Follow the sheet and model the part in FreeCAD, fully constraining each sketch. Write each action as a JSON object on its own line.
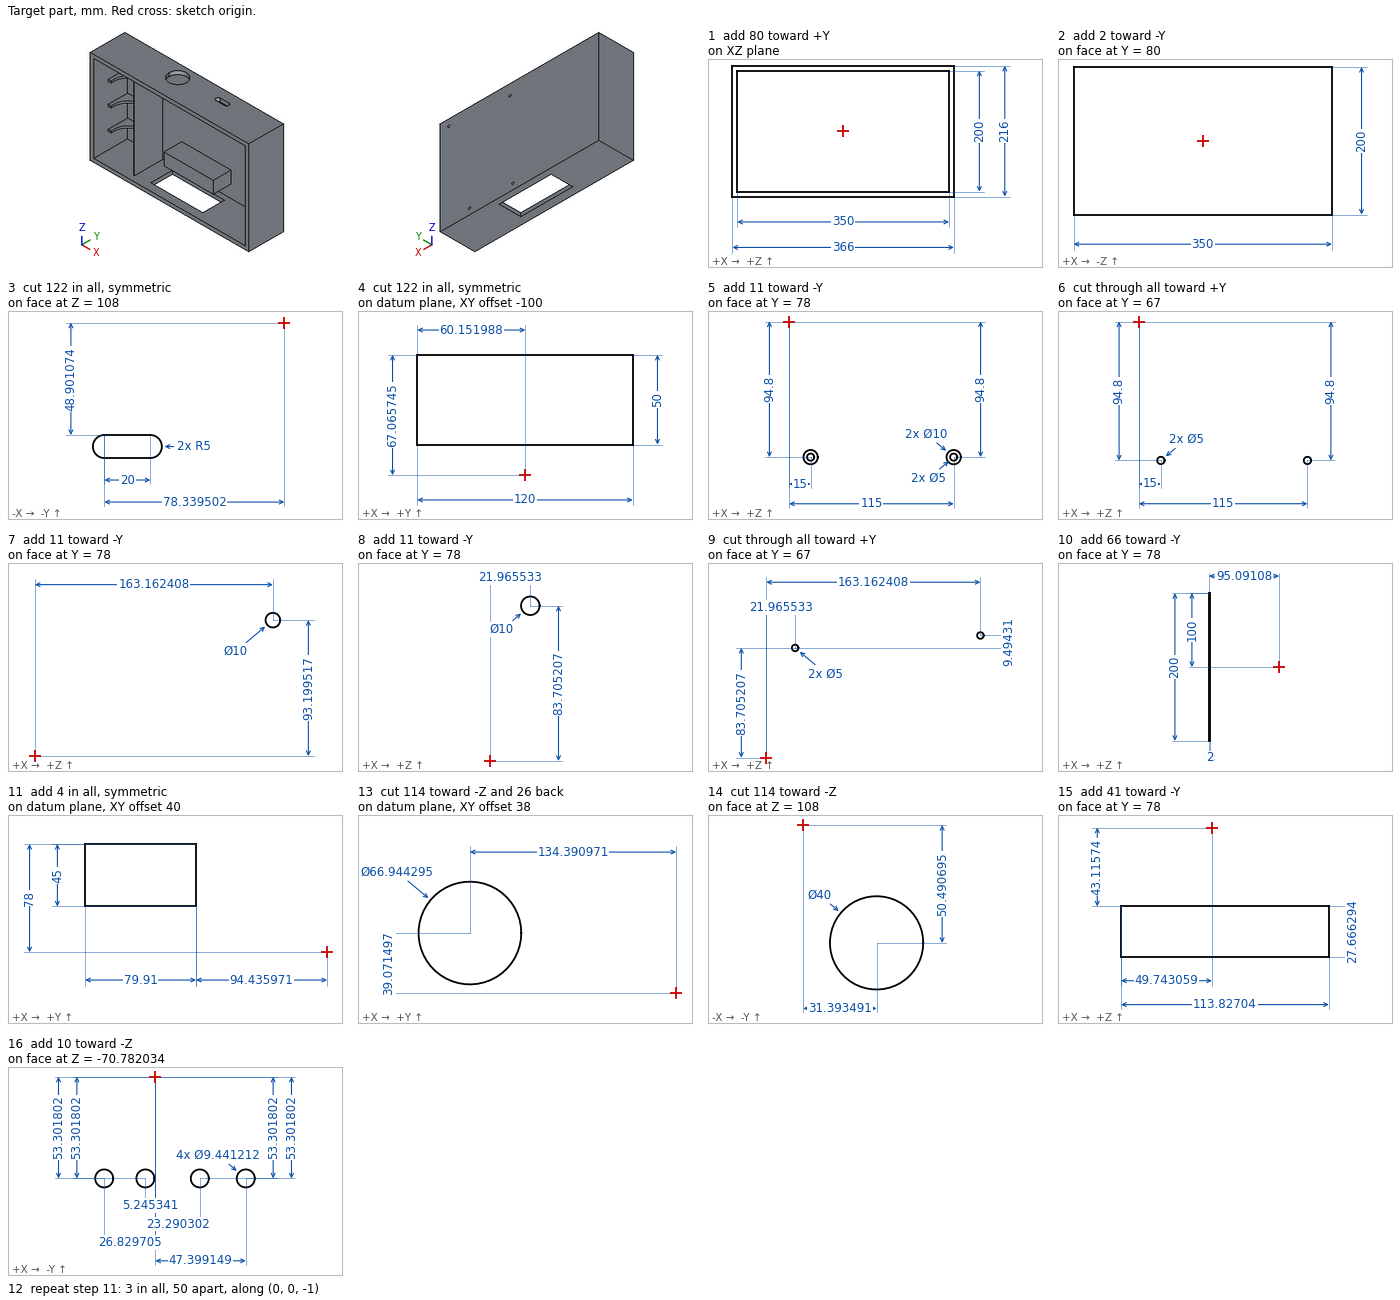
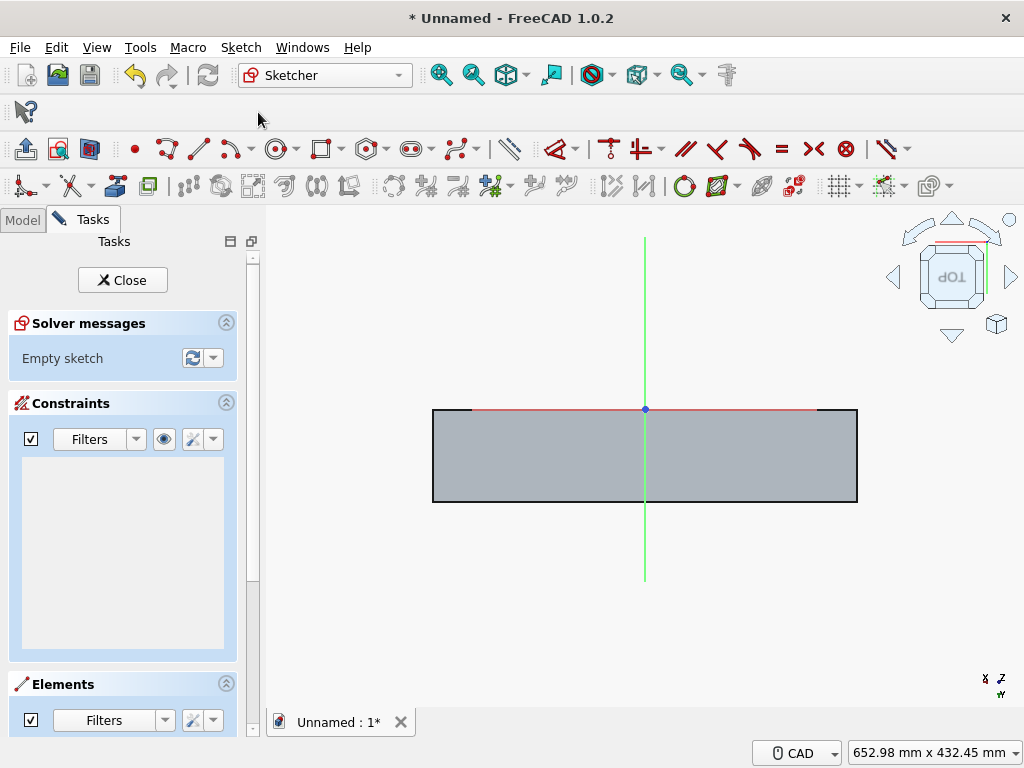
{"action": "scroll", "coordinate": [565, 474], "scroll_direction": "up", "scroll_amount": 12}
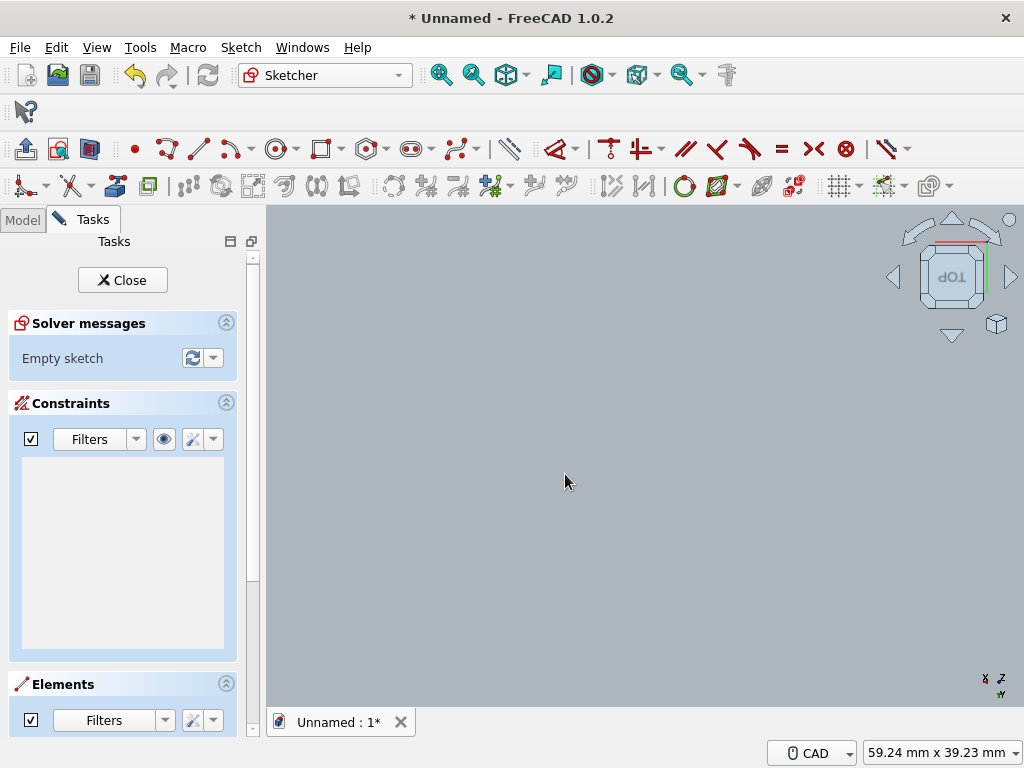
{"action": "key", "text": "g s"}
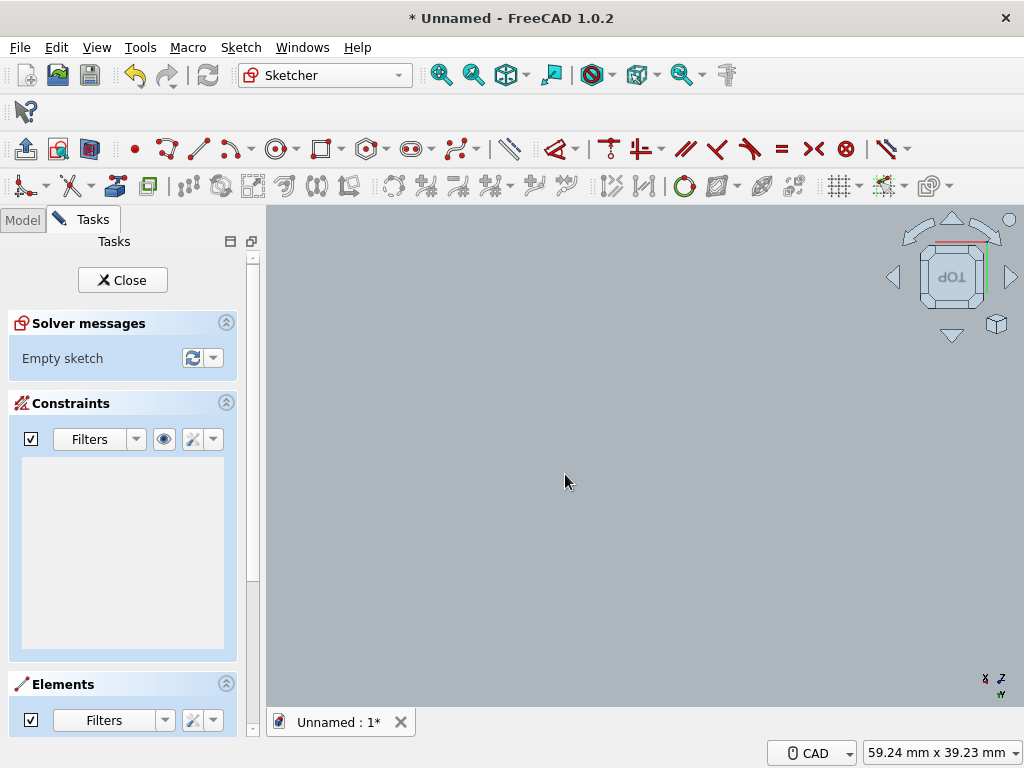
{"action": "left_click", "coordinate": [440, 448]}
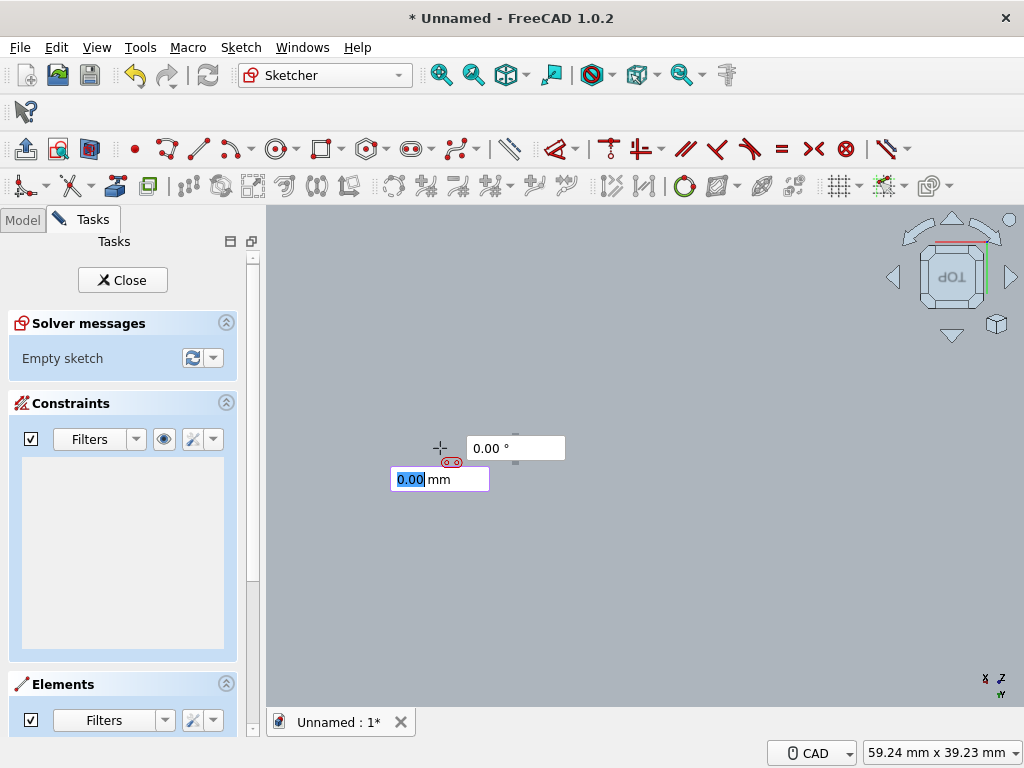
{"action": "left_click", "coordinate": [696, 448]}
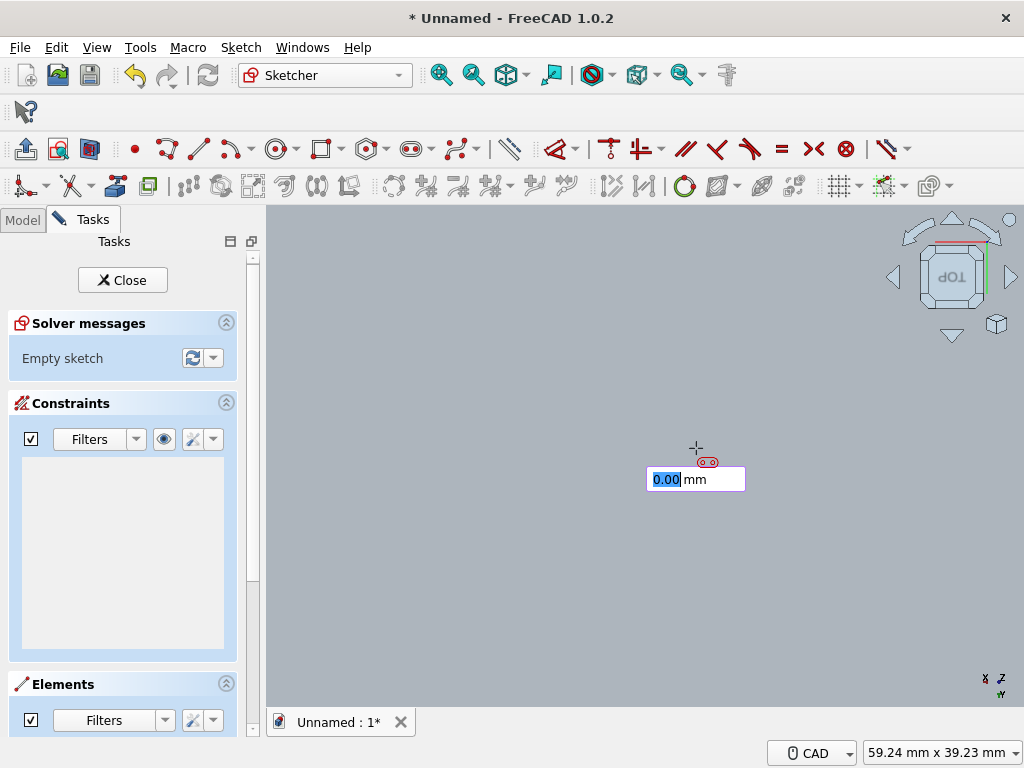
{"action": "left_click", "coordinate": [568, 512]}
{"action": "key", "text": "Escape"}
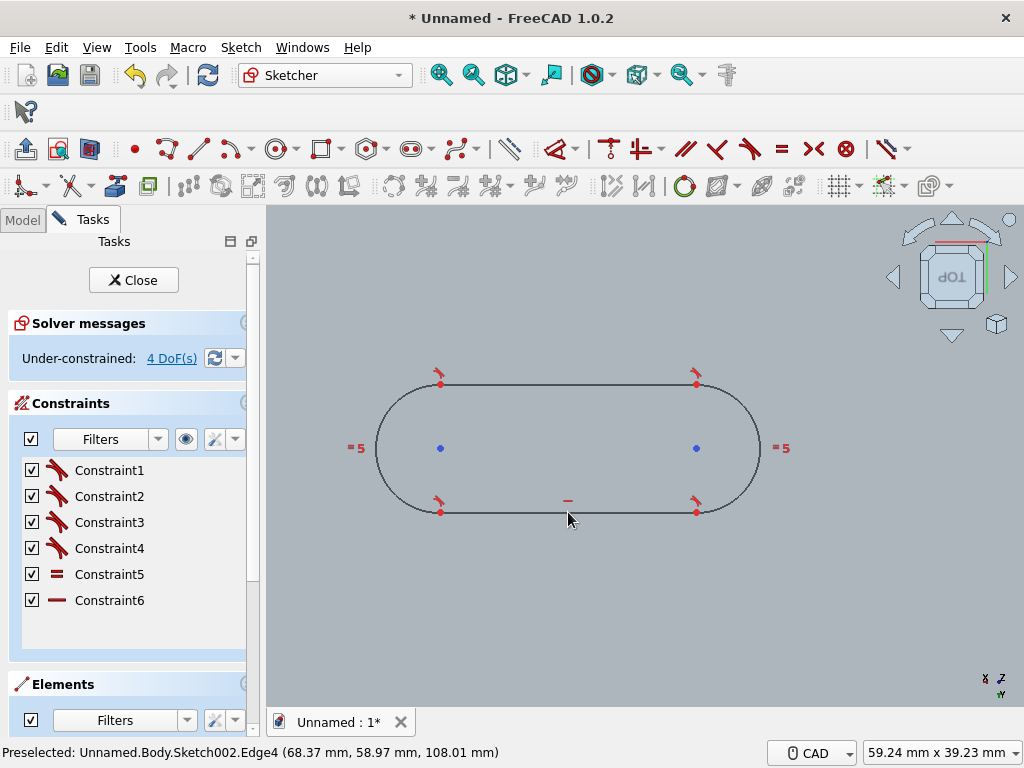
{"action": "left_click", "coordinate": [556, 150]}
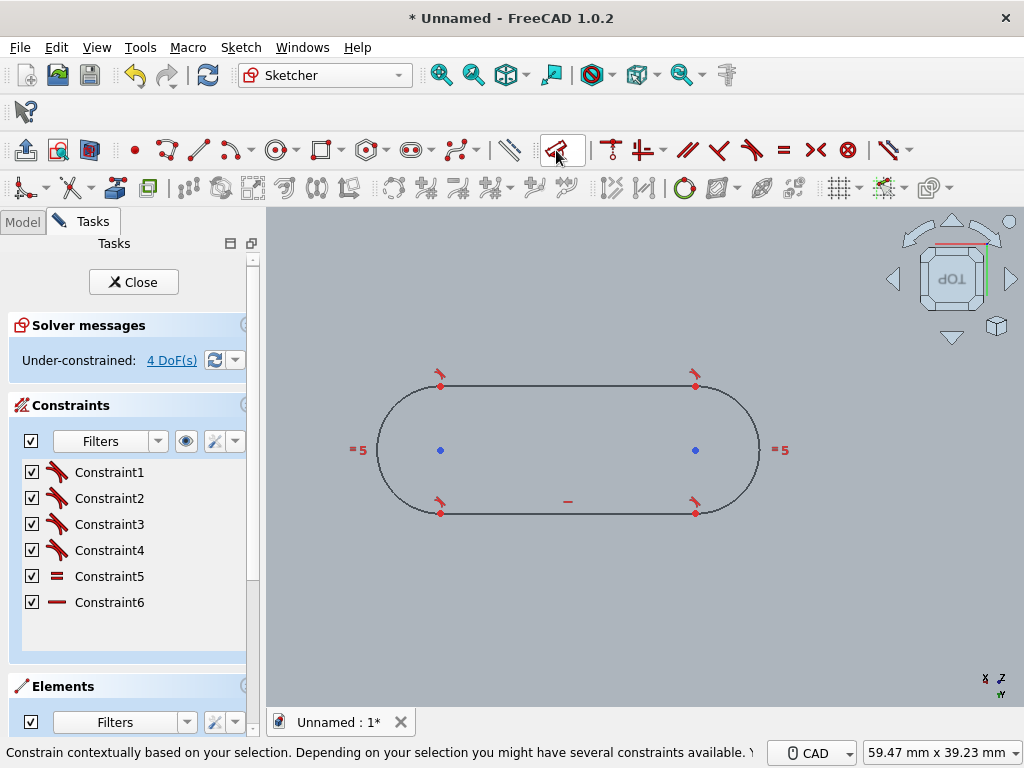
{"action": "left_click", "coordinate": [389, 413]}
{"action": "left_click", "coordinate": [363, 394]}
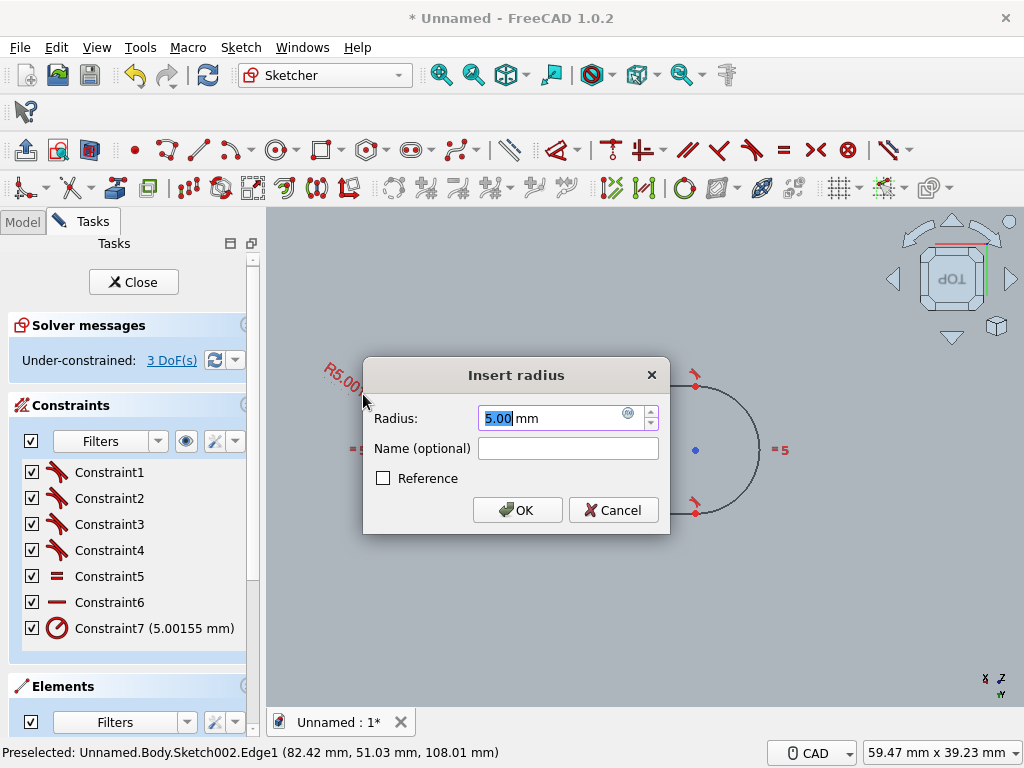
{"action": "type", "text": "5"}
{"action": "key", "text": "Return"}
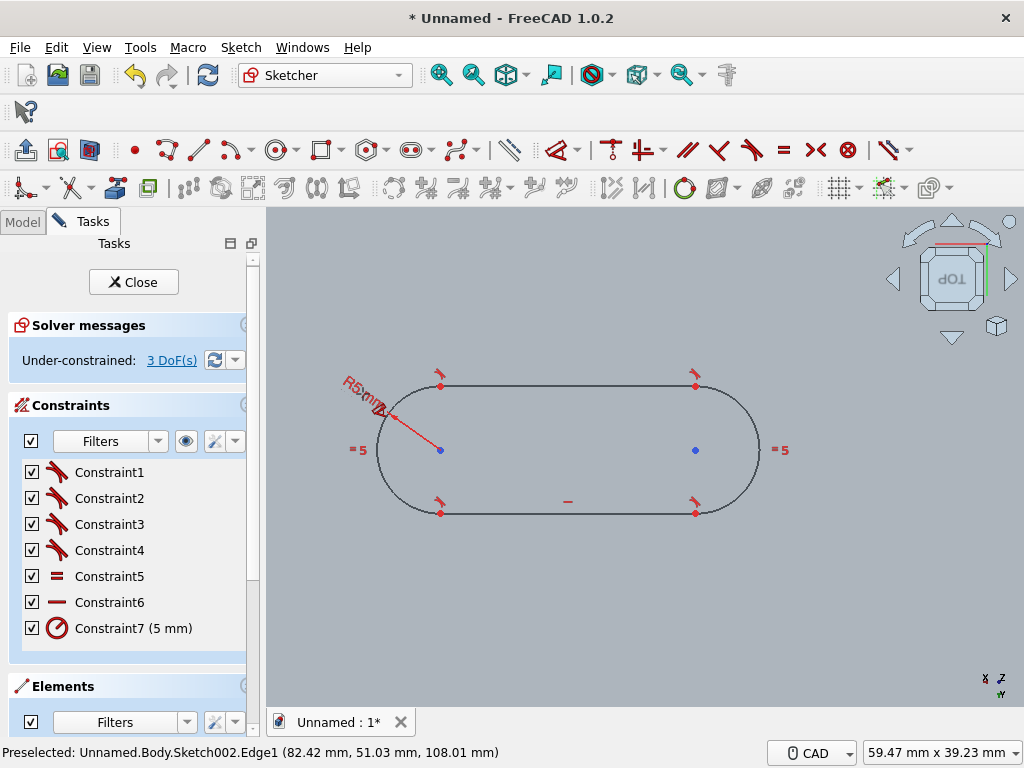
{"action": "left_click", "coordinate": [517, 386]}
{"action": "left_click", "coordinate": [568, 352]}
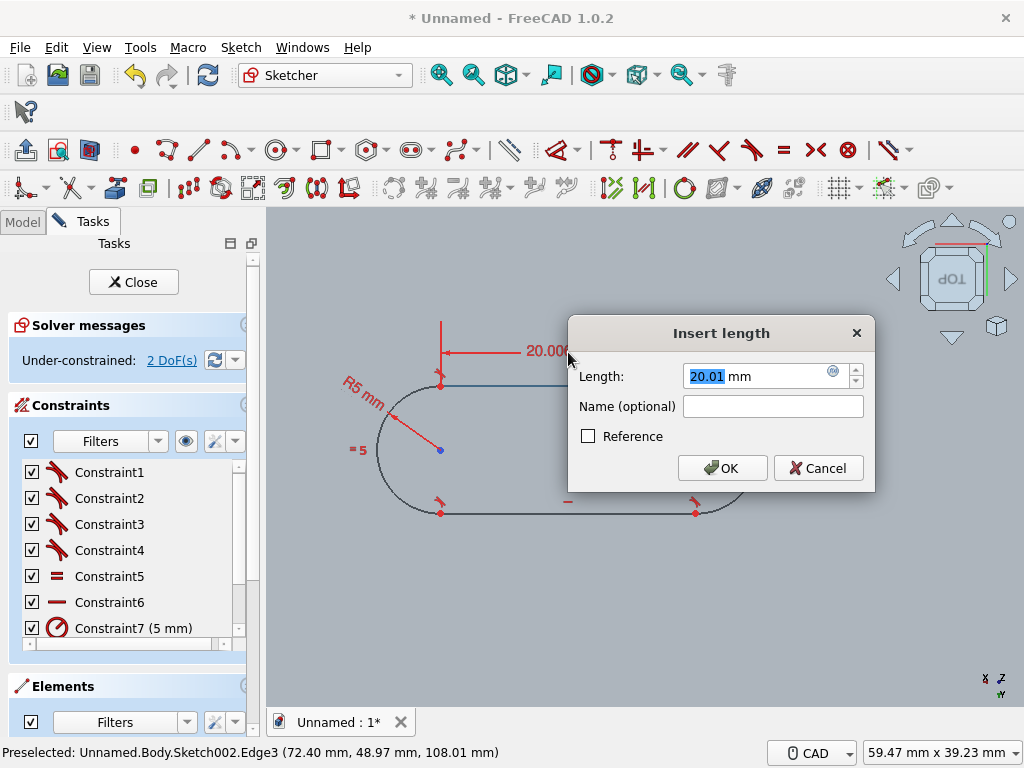
{"action": "type", "text": "20"}
{"action": "key", "text": "Return"}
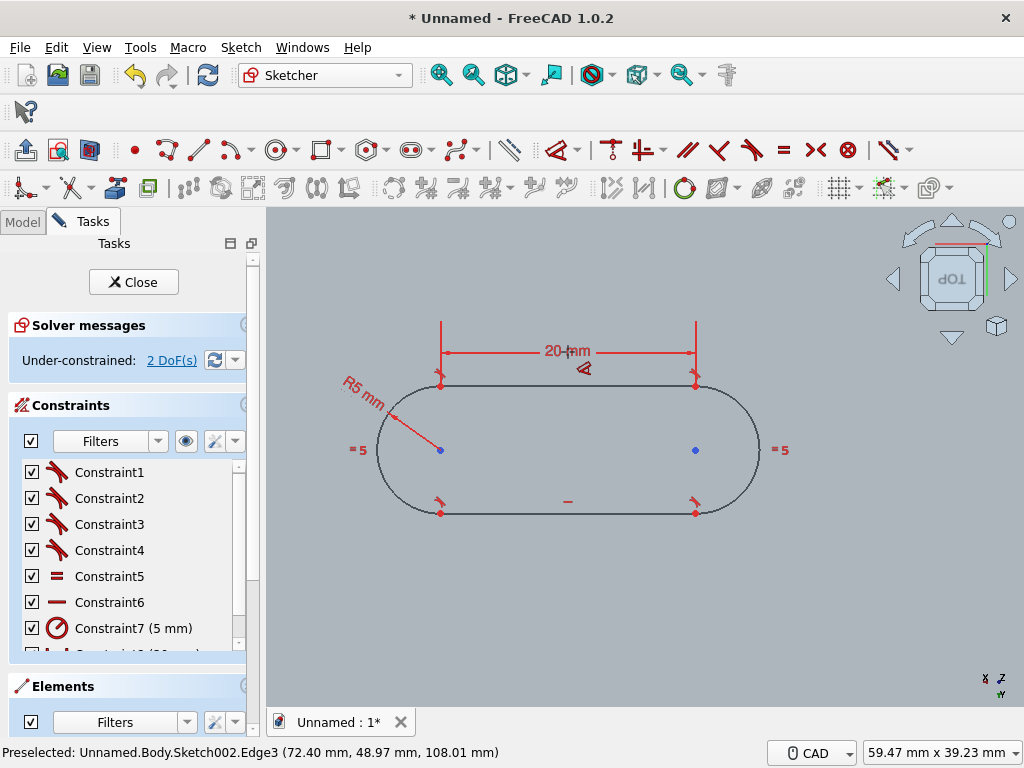
{"action": "left_click", "coordinate": [441, 386]}
{"action": "left_click", "coordinate": [650, 420]}